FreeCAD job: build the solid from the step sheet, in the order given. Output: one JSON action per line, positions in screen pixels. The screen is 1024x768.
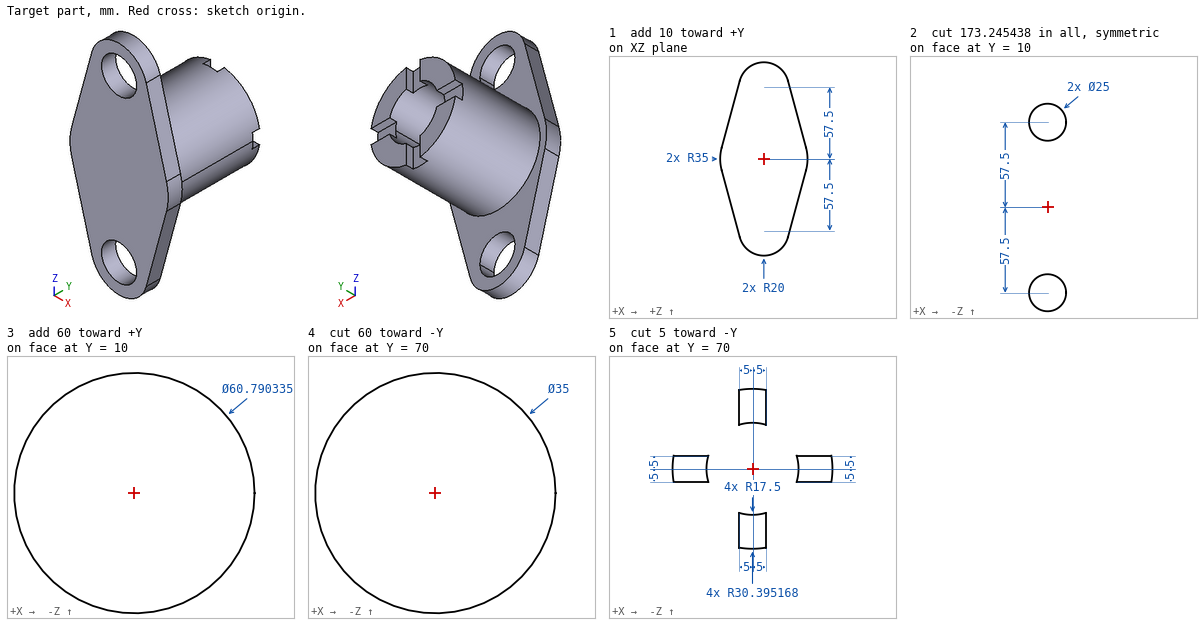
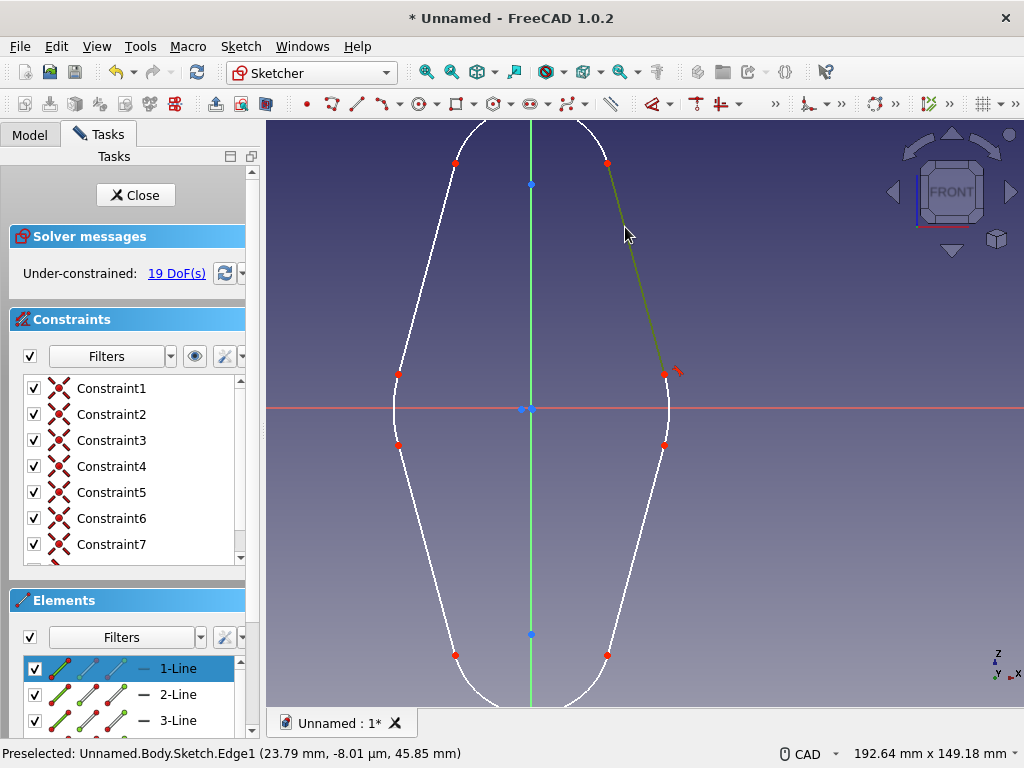
{"action": "scroll", "coordinate": [668, 424], "scroll_direction": "down", "scroll_amount": 2}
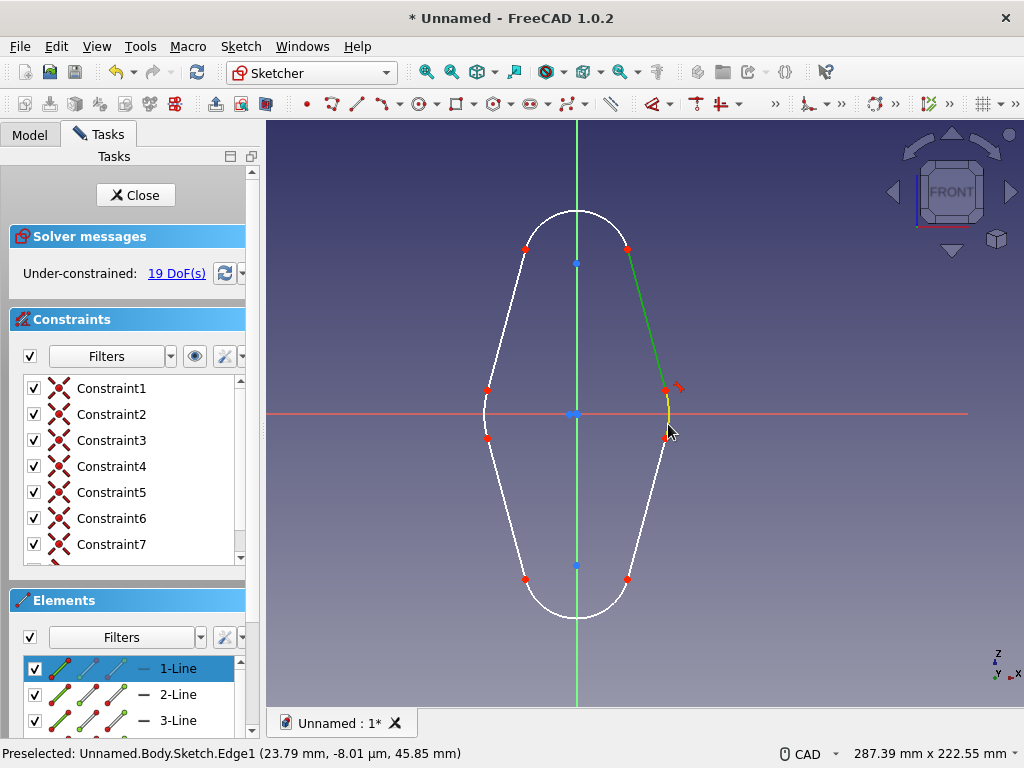
{"action": "left_click", "coordinate": [603, 218]}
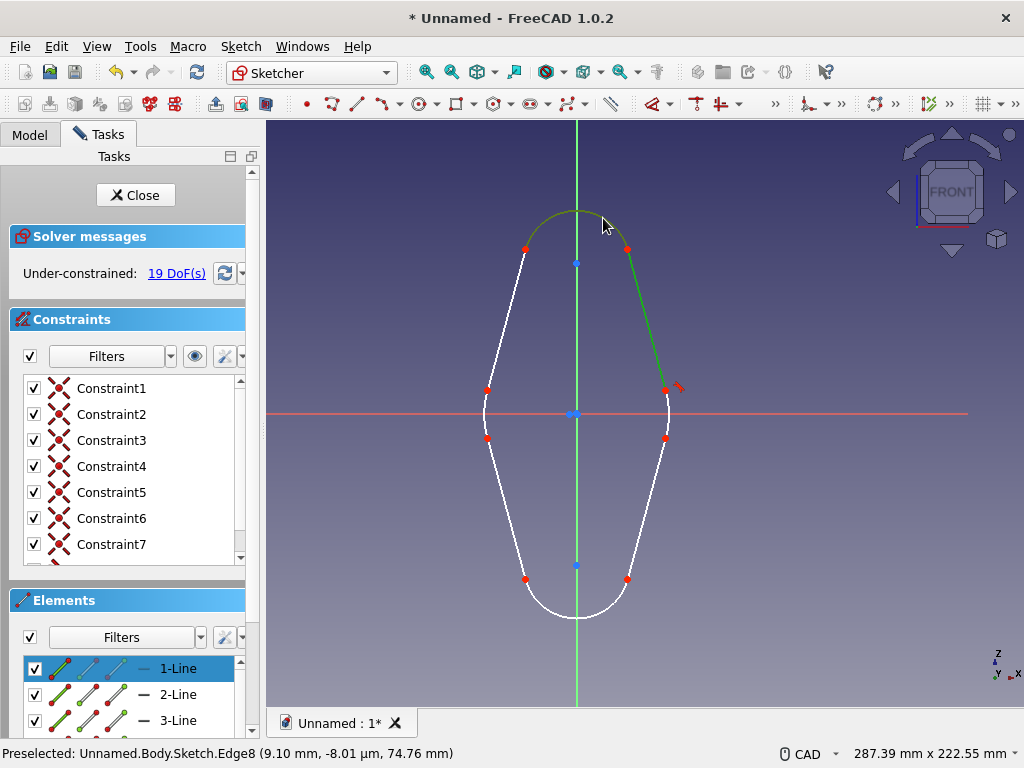
{"action": "key", "text": "t"}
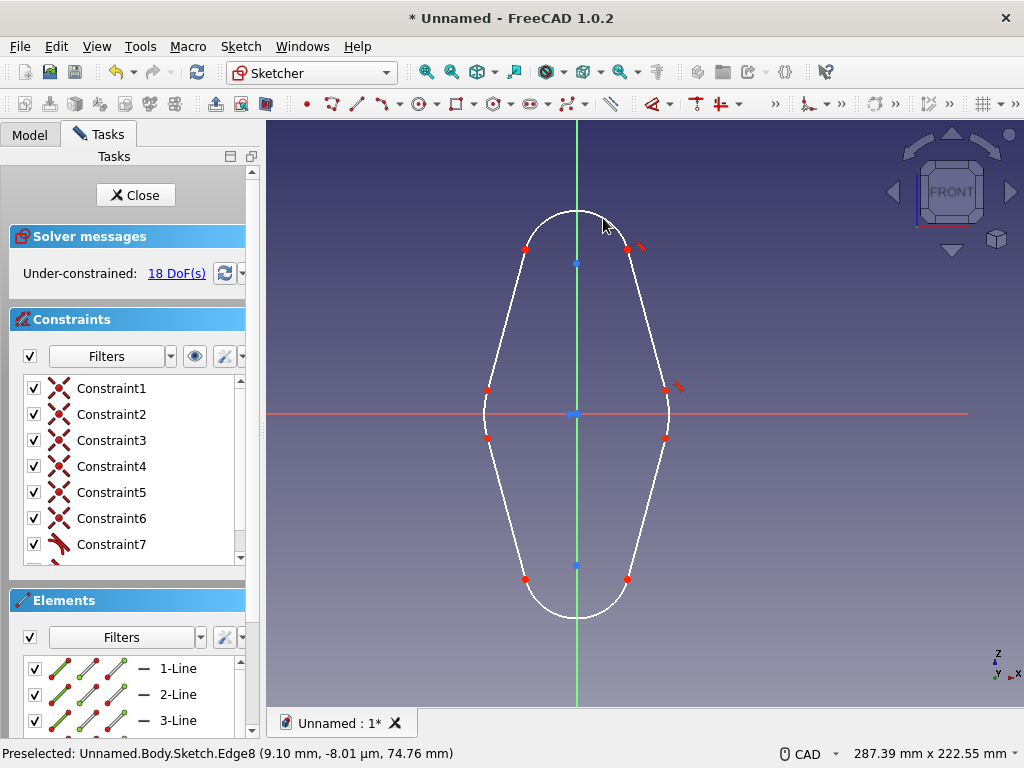
{"action": "left_click", "coordinate": [654, 481]}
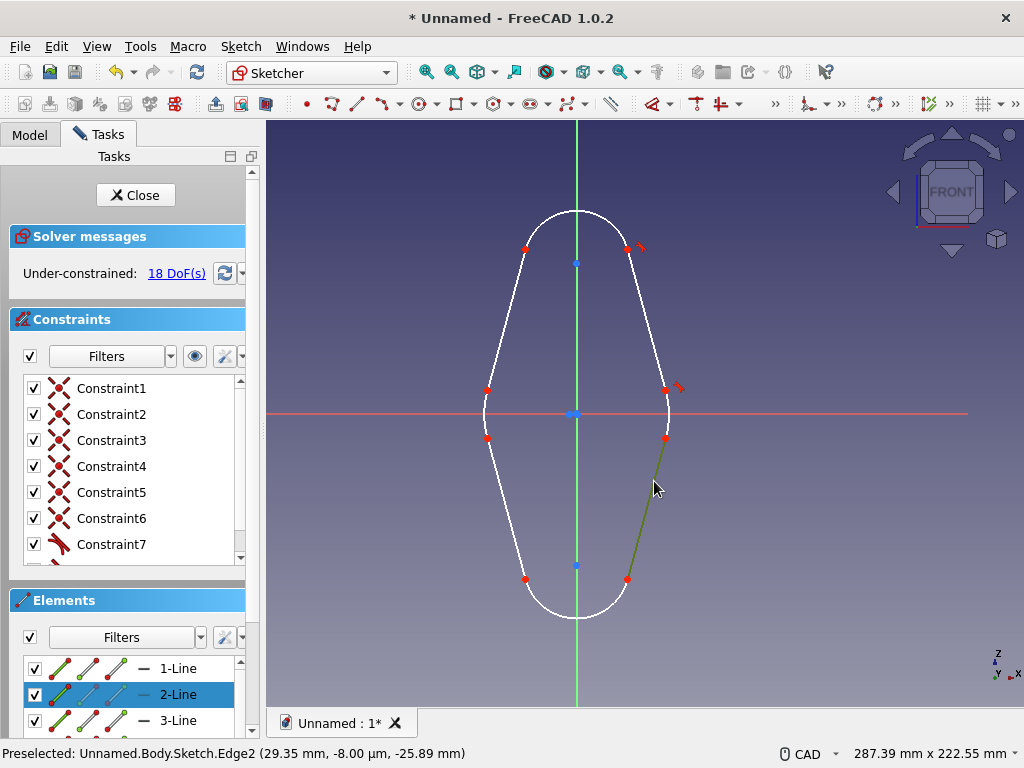
{"action": "scroll", "coordinate": [668, 424], "scroll_direction": "up", "scroll_amount": 2}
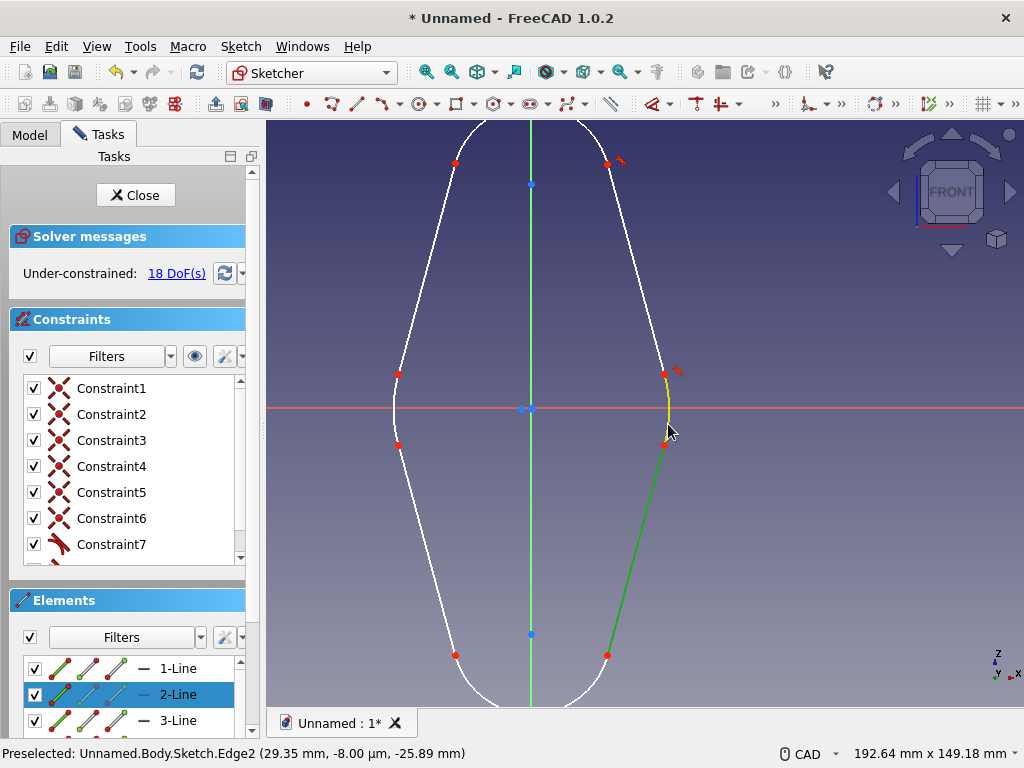
{"action": "left_click", "coordinate": [668, 424]}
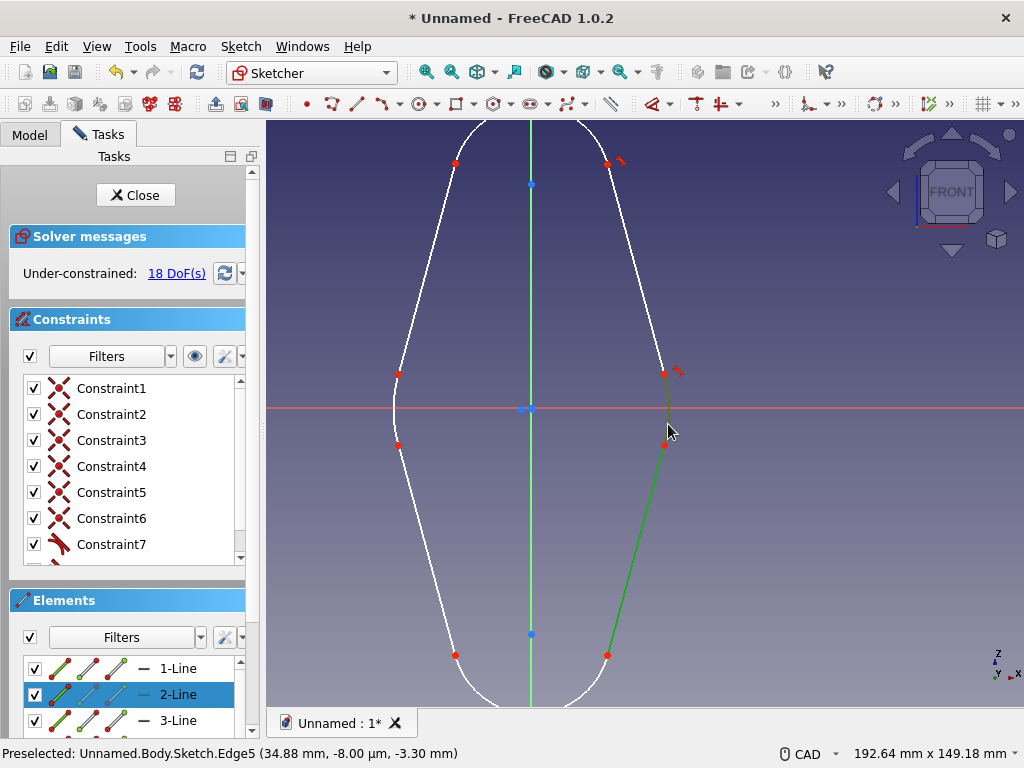
{"action": "key", "text": "t"}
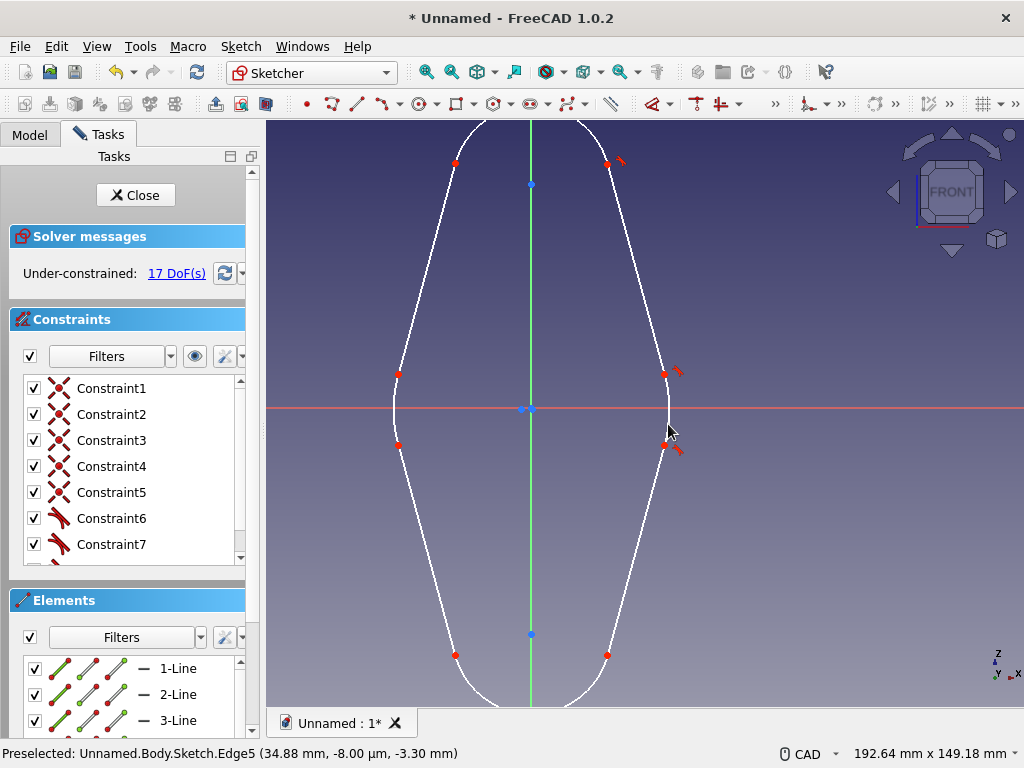
{"action": "left_click", "coordinate": [647, 509]}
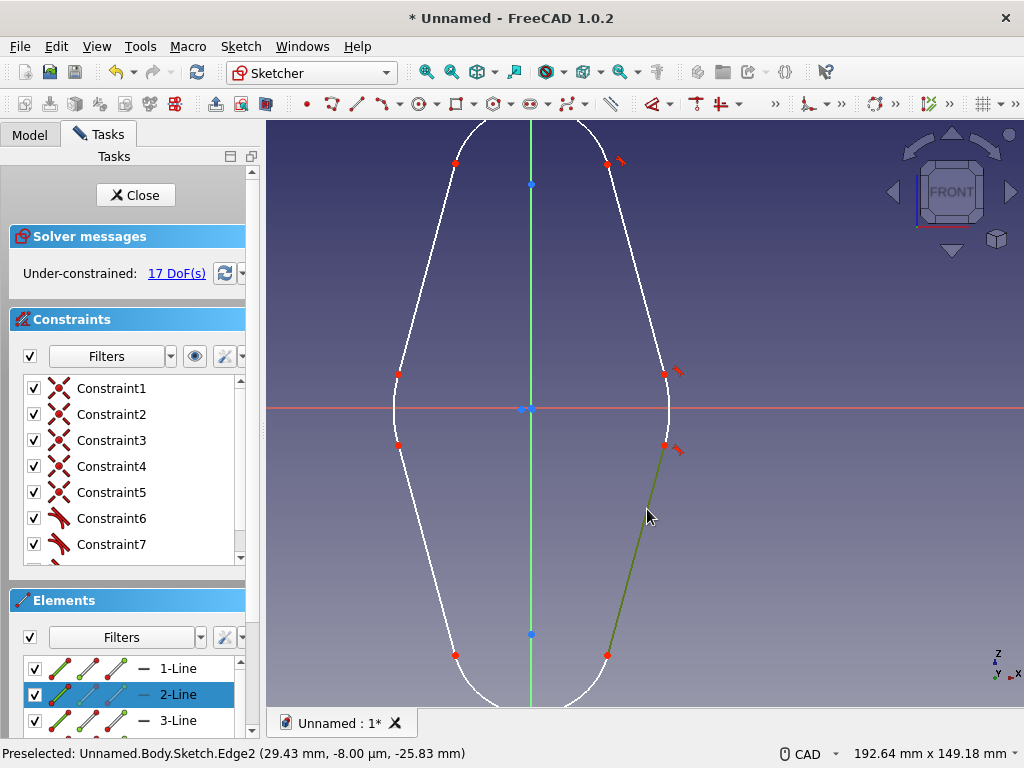
{"action": "scroll", "coordinate": [668, 424], "scroll_direction": "down", "scroll_amount": 2}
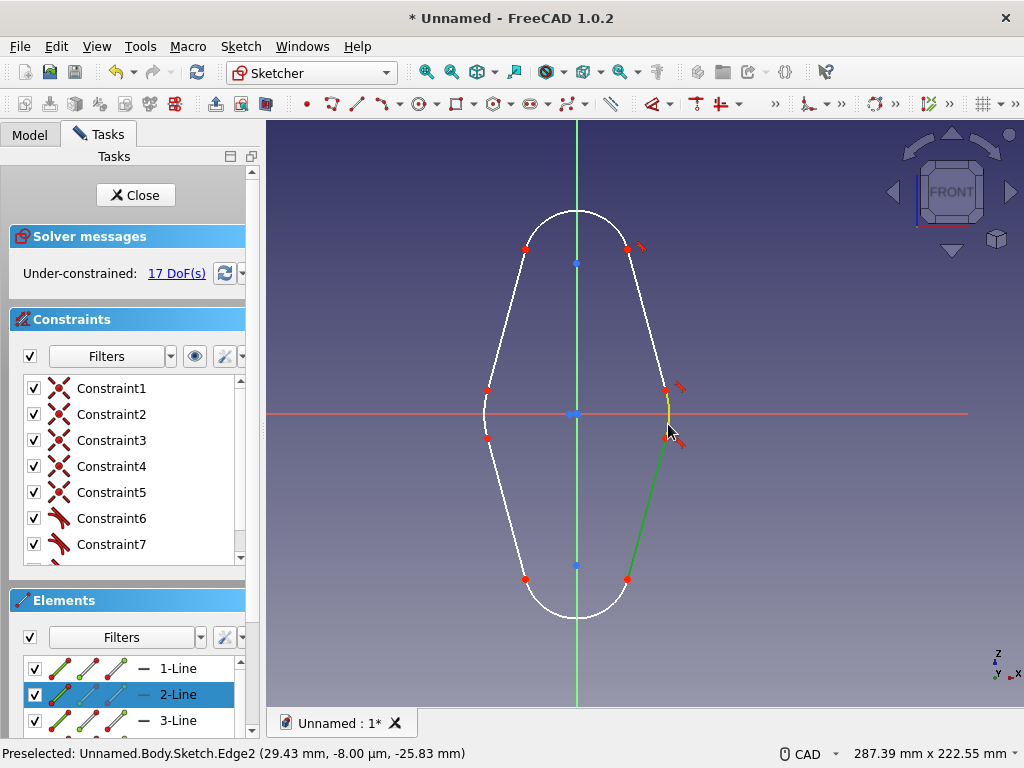
{"action": "left_click", "coordinate": [550, 611]}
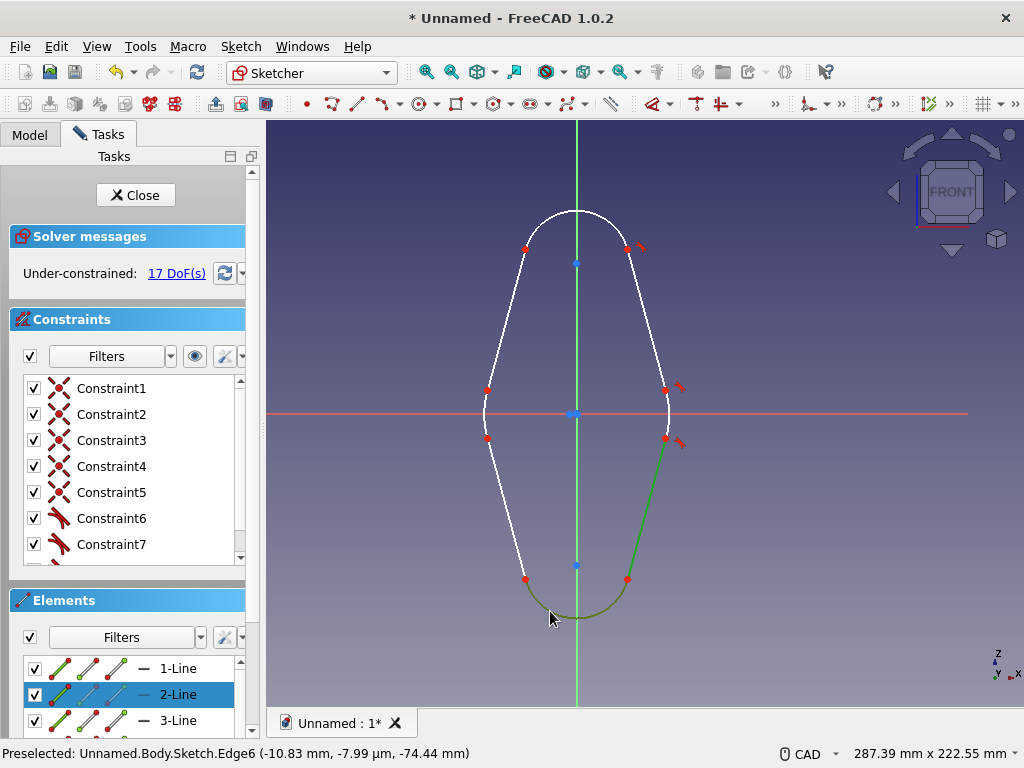
{"action": "key", "text": "t"}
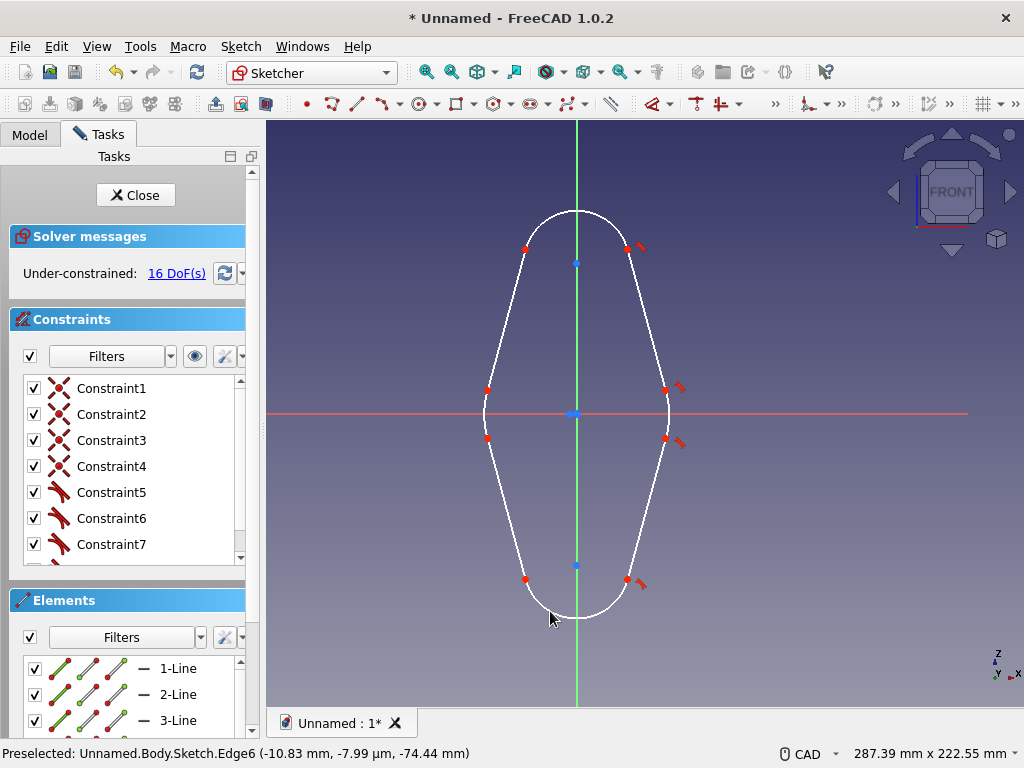
{"action": "left_click", "coordinate": [514, 537]}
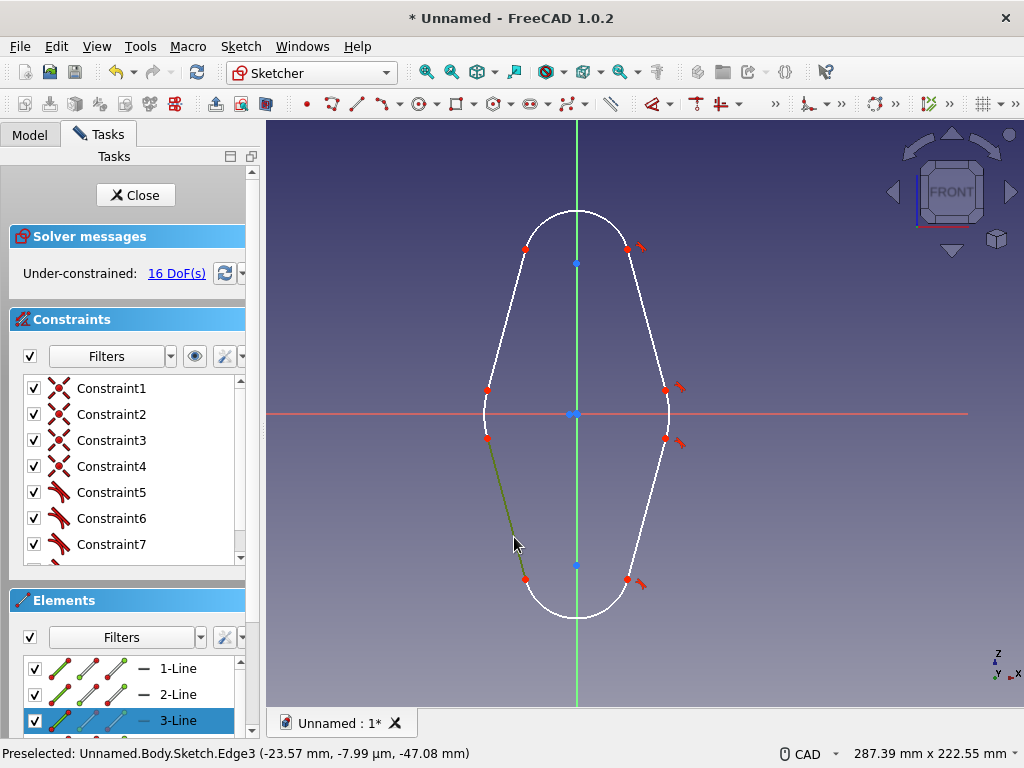
{"action": "left_click", "coordinate": [550, 612]}